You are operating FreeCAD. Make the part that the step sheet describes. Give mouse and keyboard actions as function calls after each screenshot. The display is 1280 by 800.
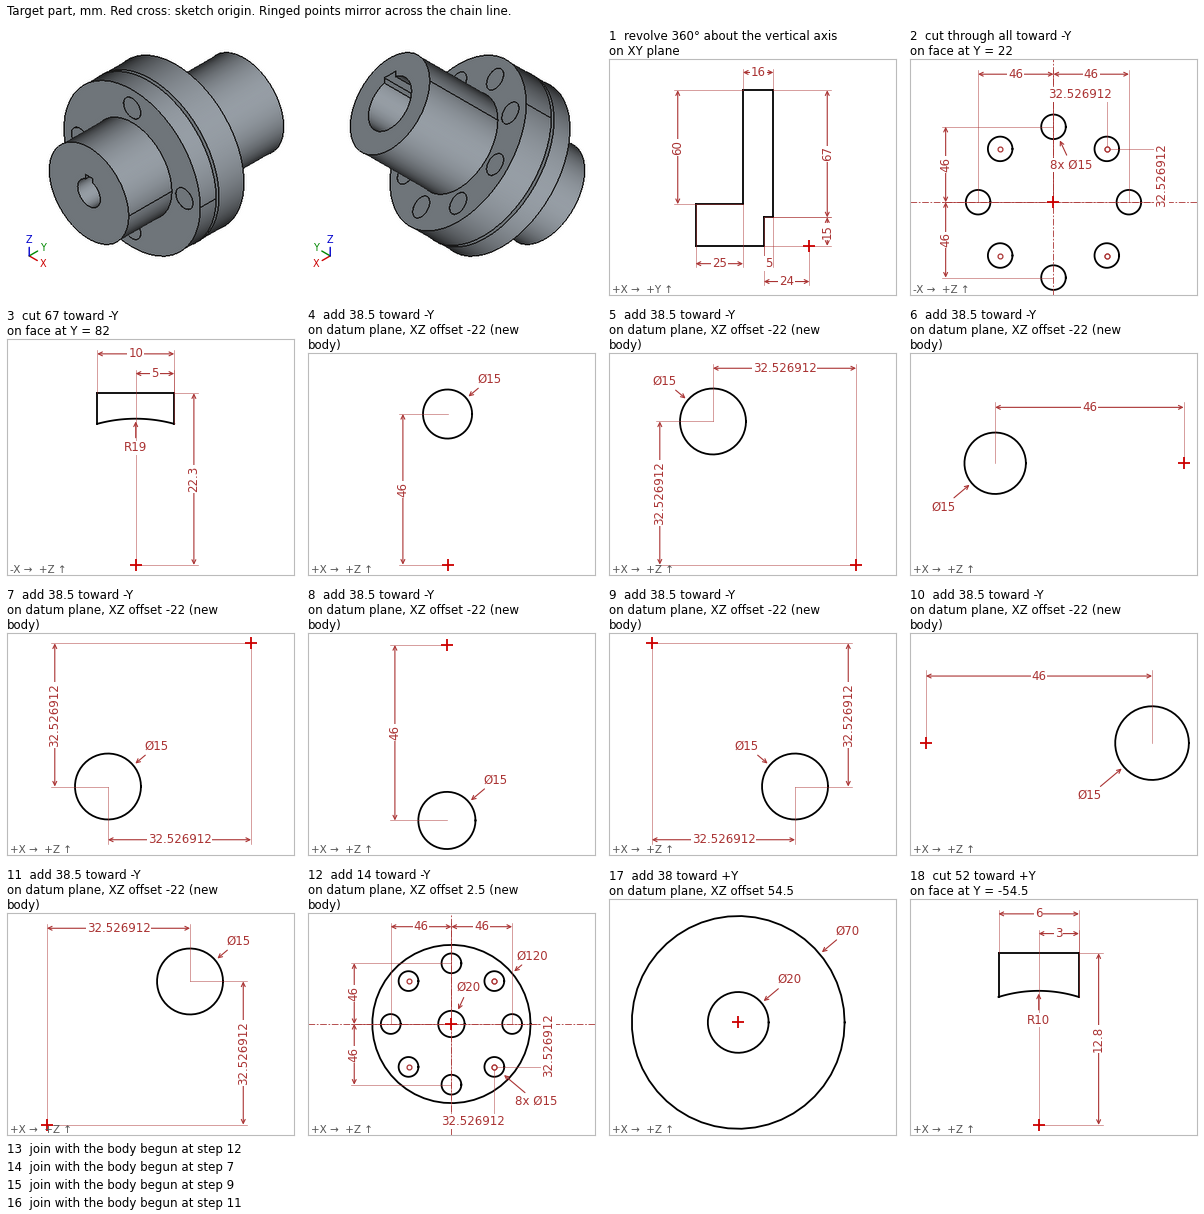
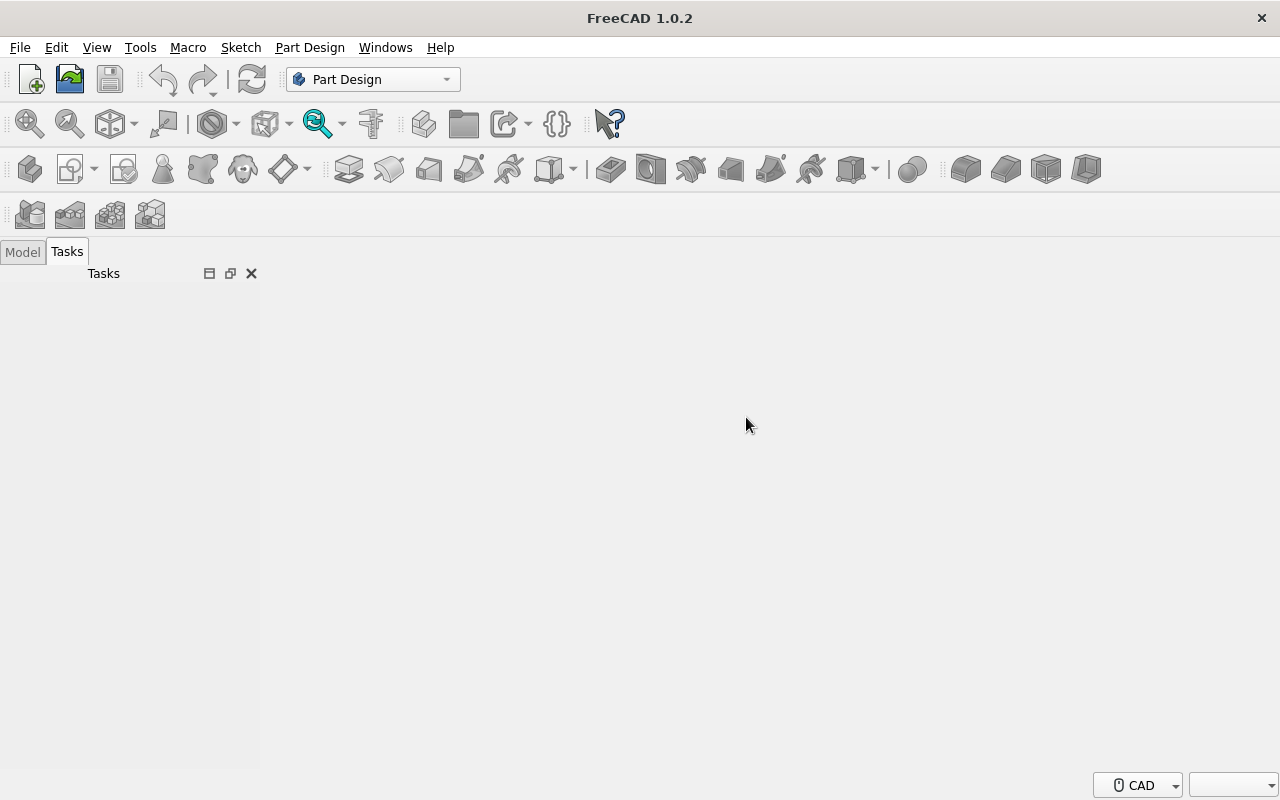
click(30, 80)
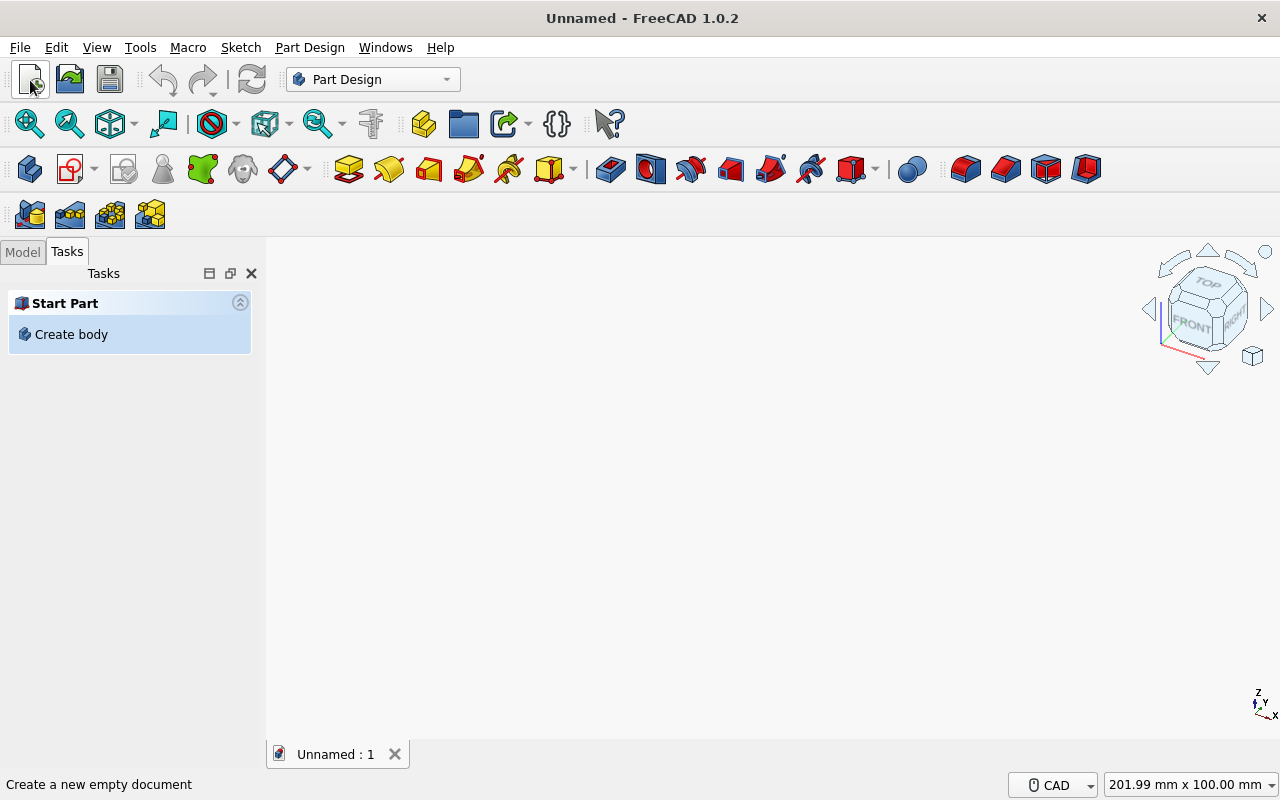
click(70, 170)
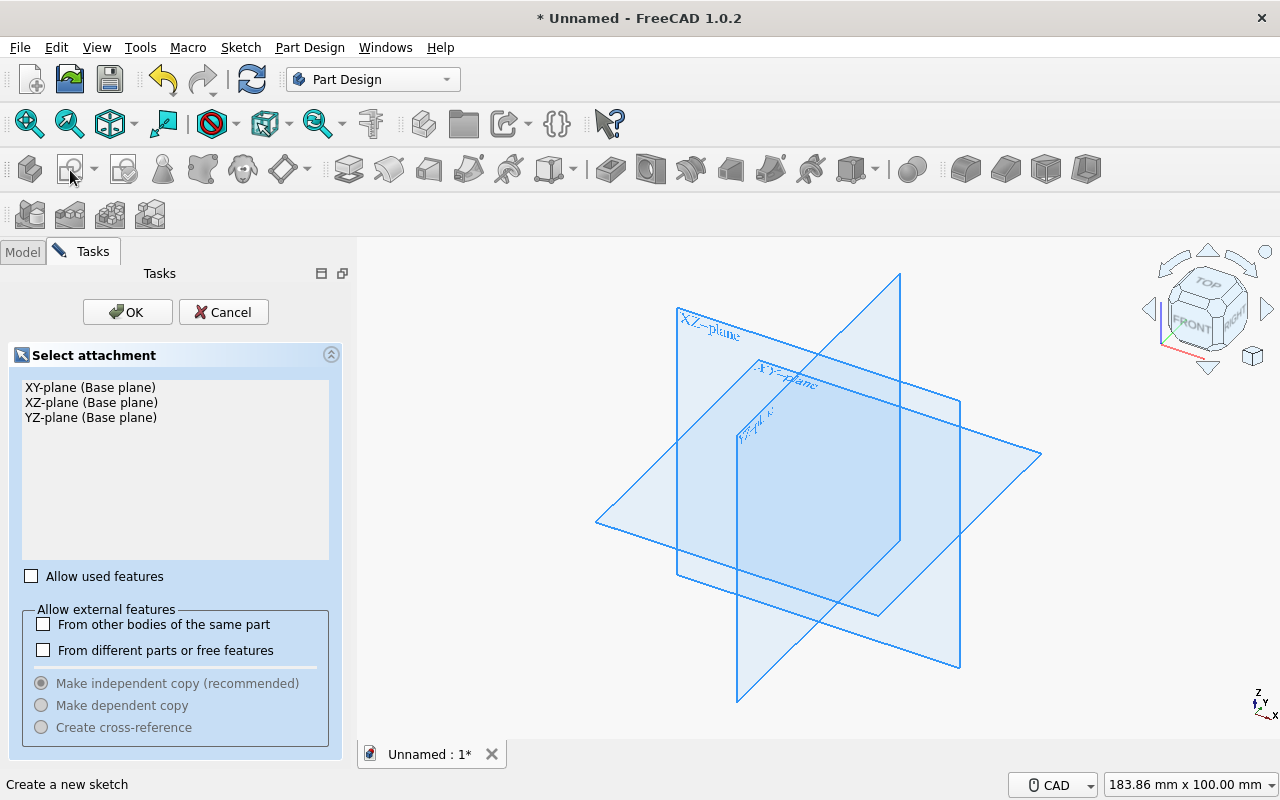
click(82, 388)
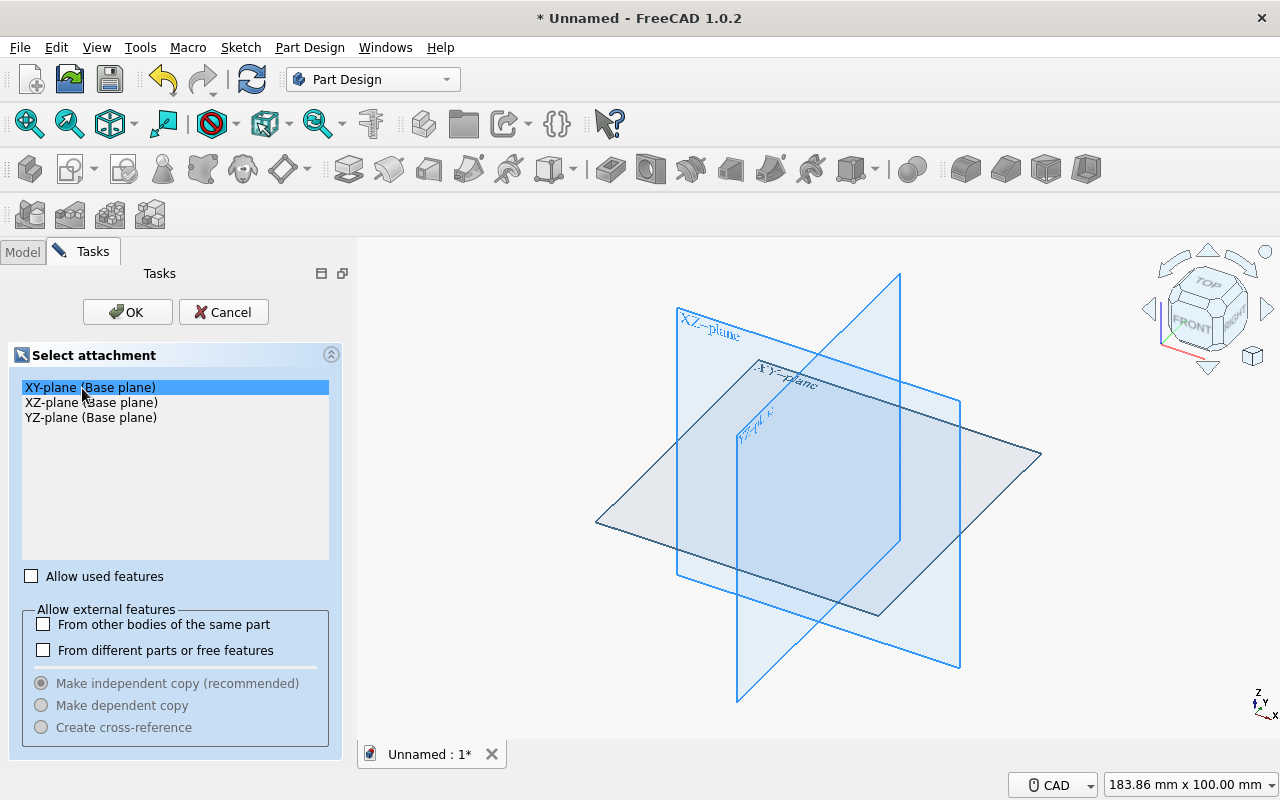
click(128, 312)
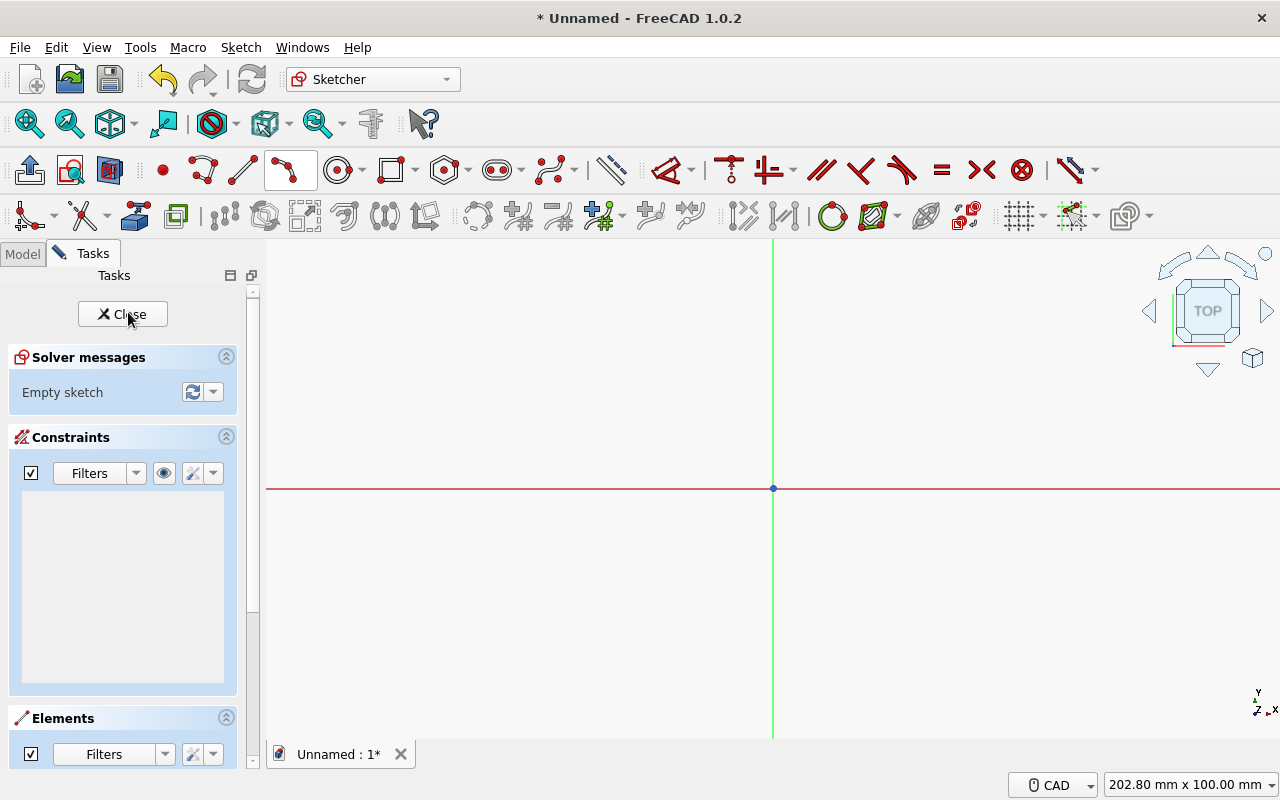
scroll(804, 711, down, 3)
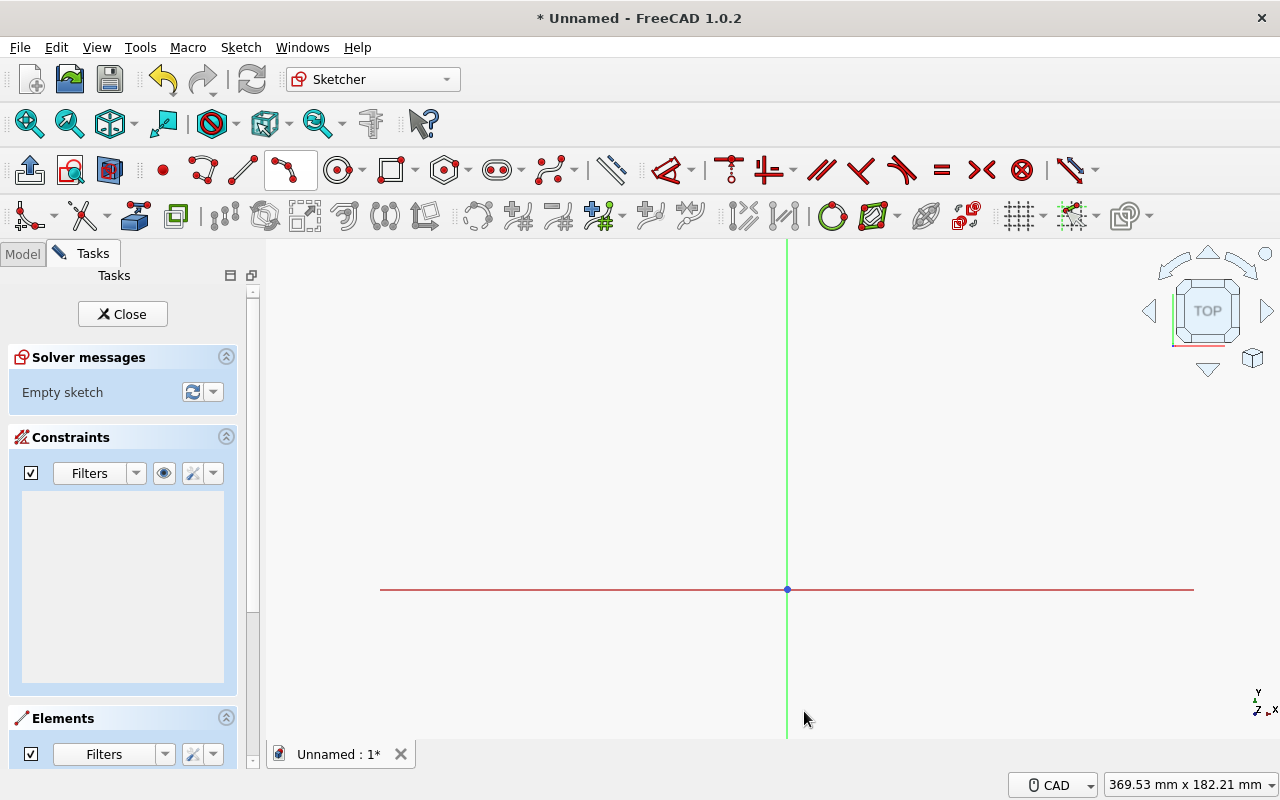
scroll(706, 453, up, 2)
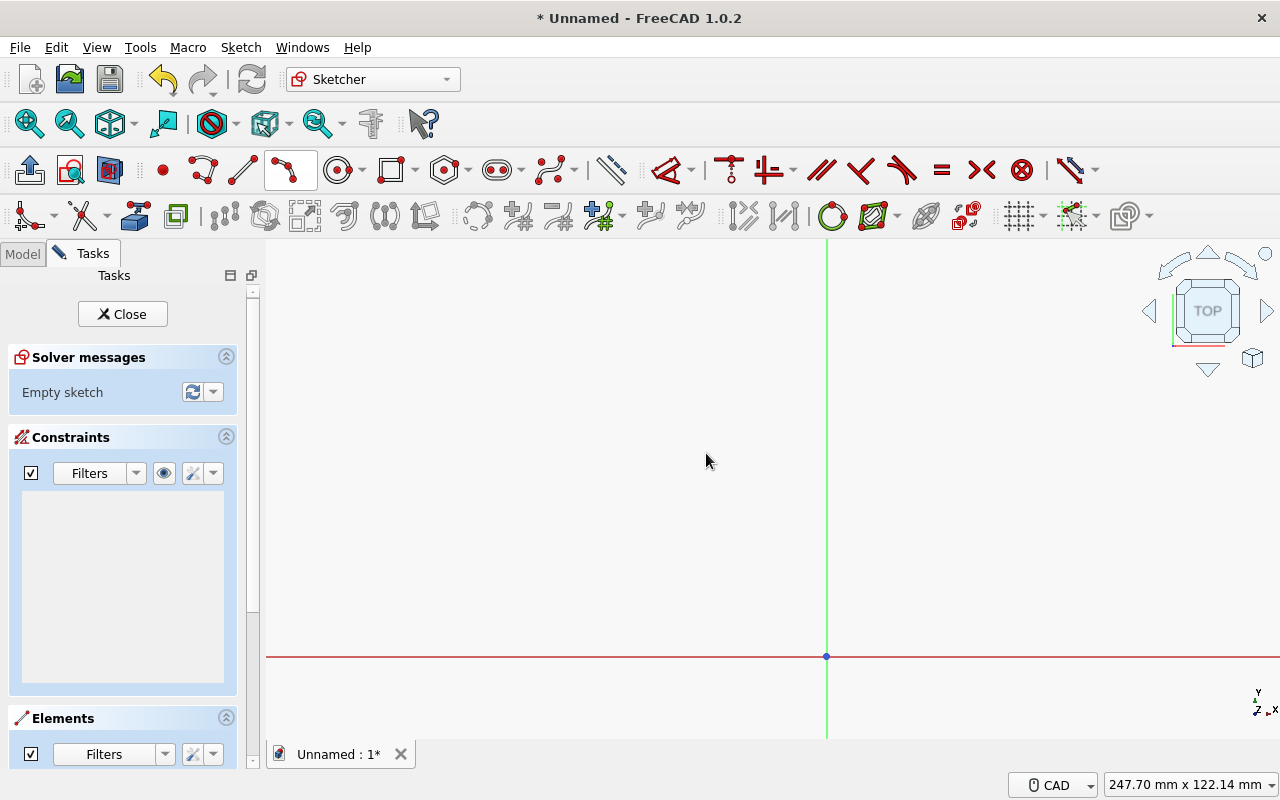
click(204, 170)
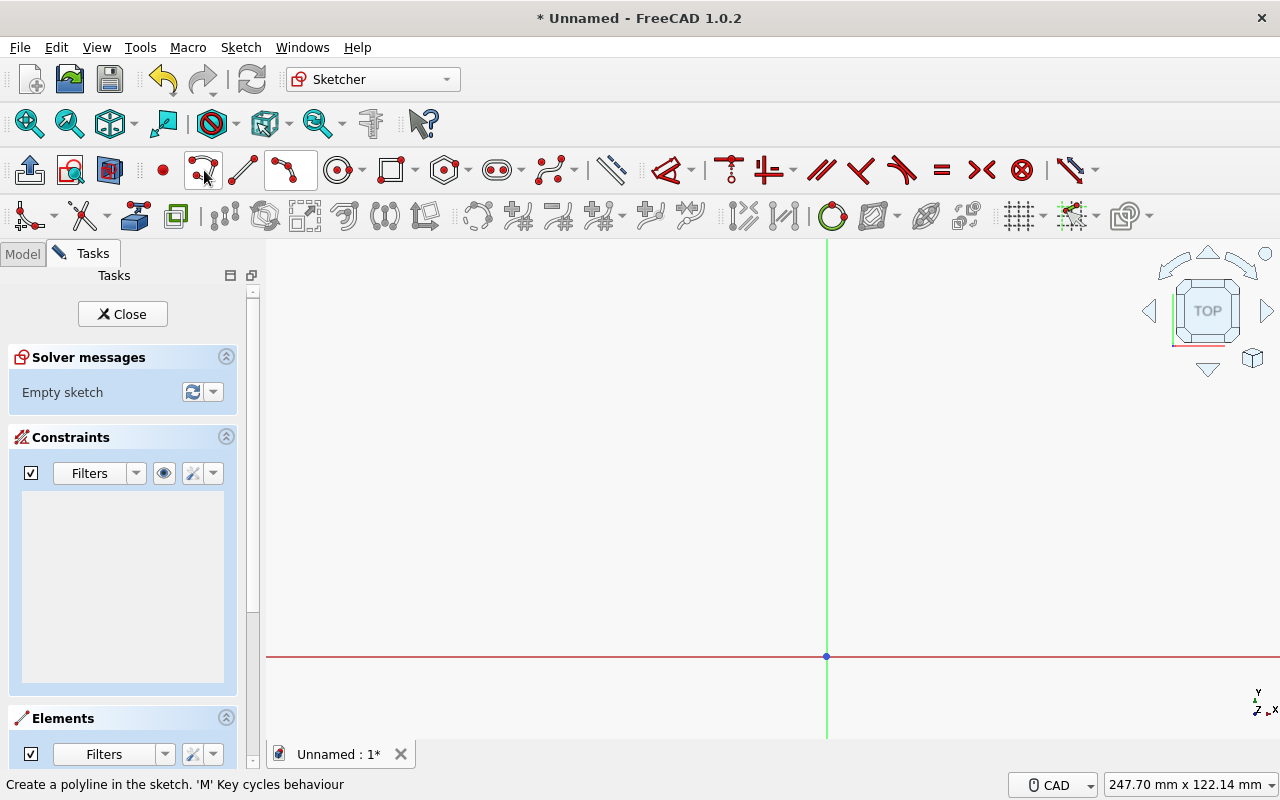
click(729, 657)
click(729, 595)
click(749, 595)
click(749, 321)
click(684, 321)
click(684, 566)
click(581, 566)
click(581, 648)
click(729, 657)
key(Escape)
key(Escape)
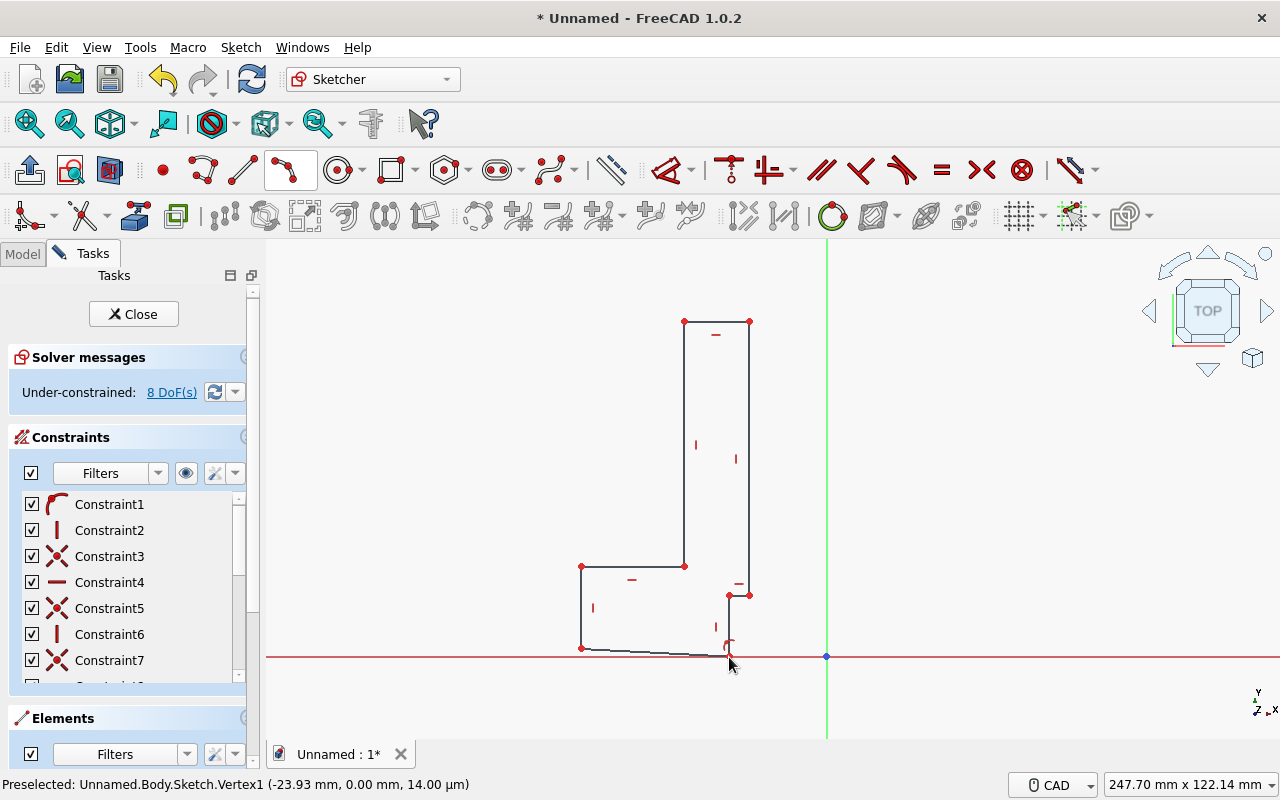
click(685, 654)